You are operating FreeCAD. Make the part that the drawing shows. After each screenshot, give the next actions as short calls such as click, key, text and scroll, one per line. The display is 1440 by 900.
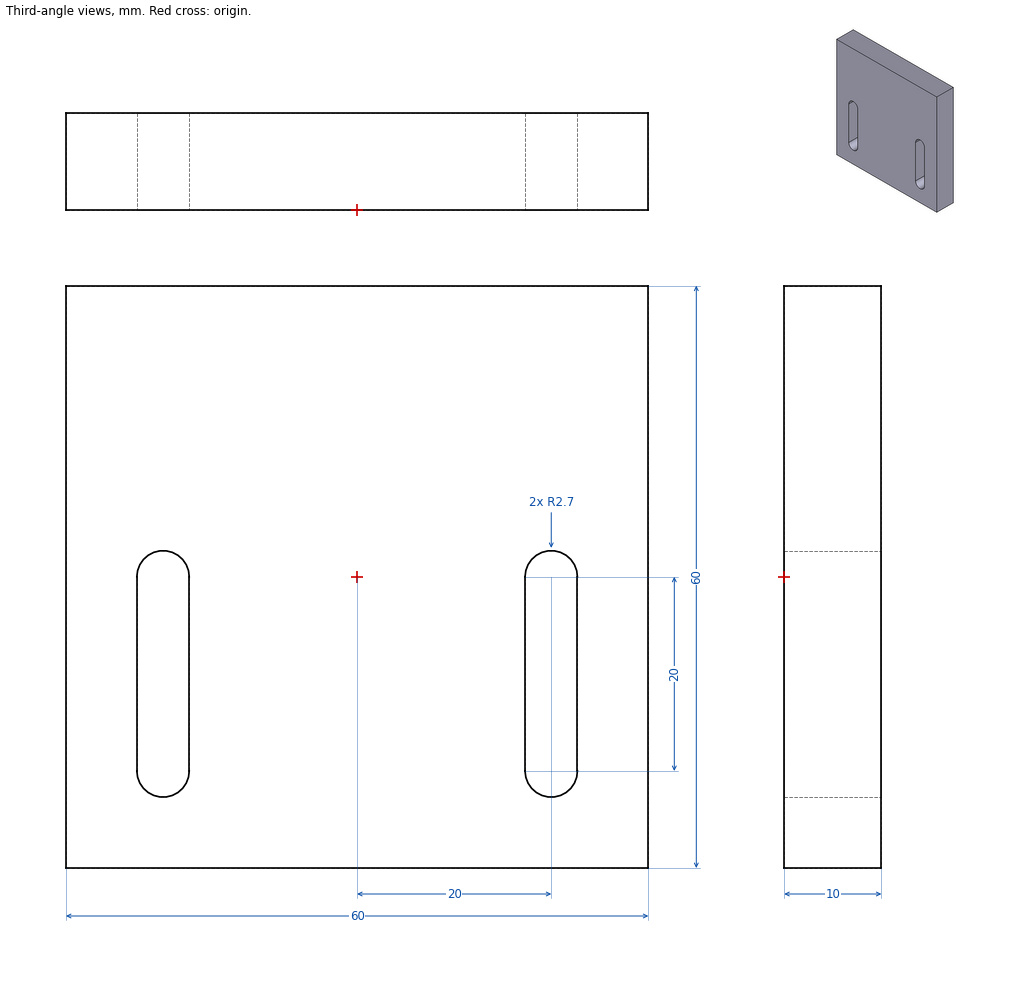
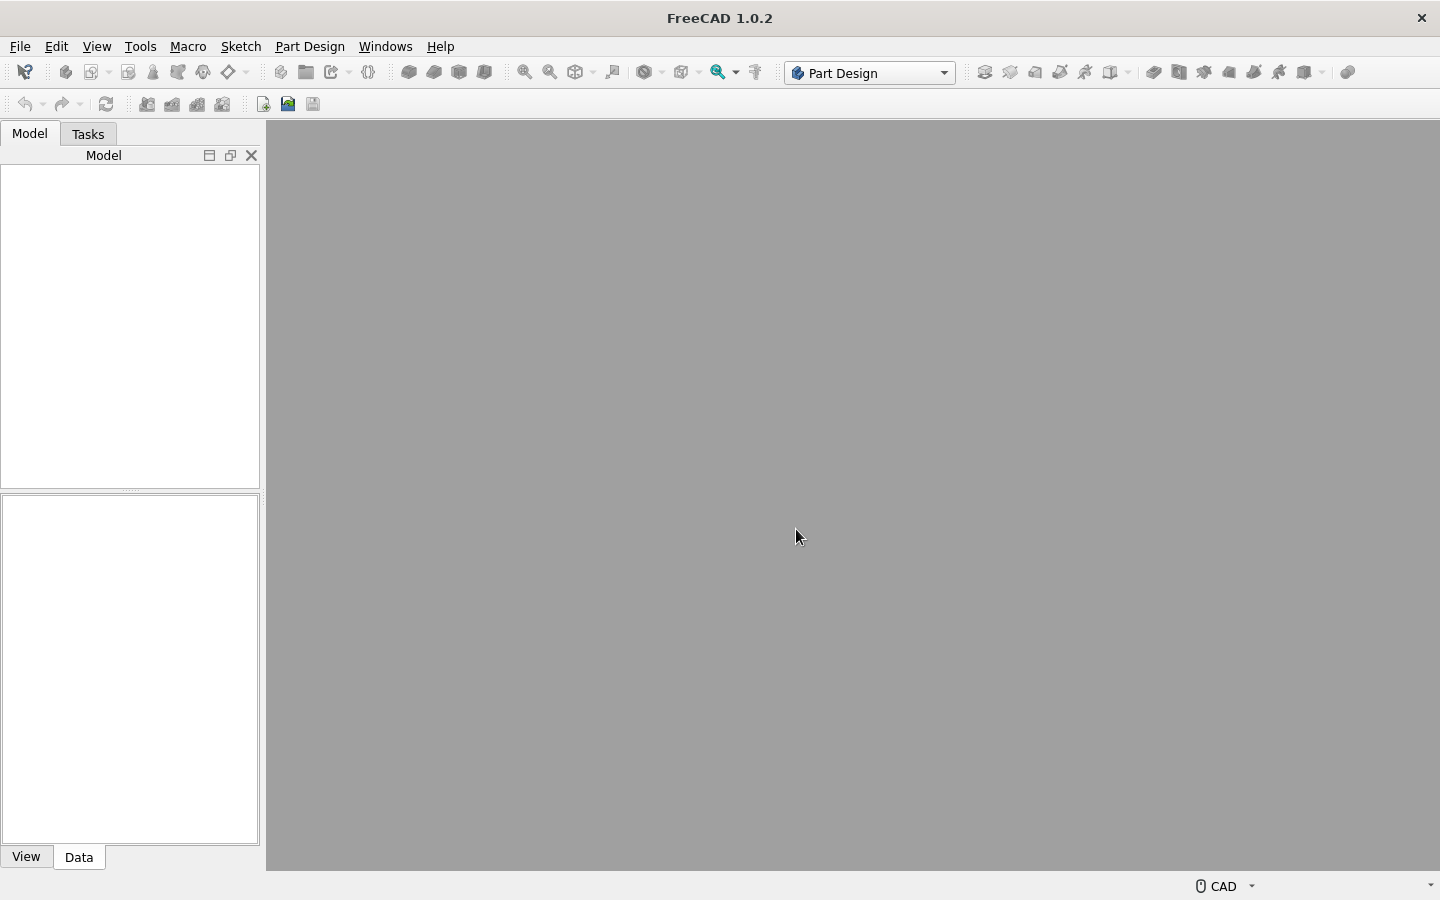
key(ctrl+n)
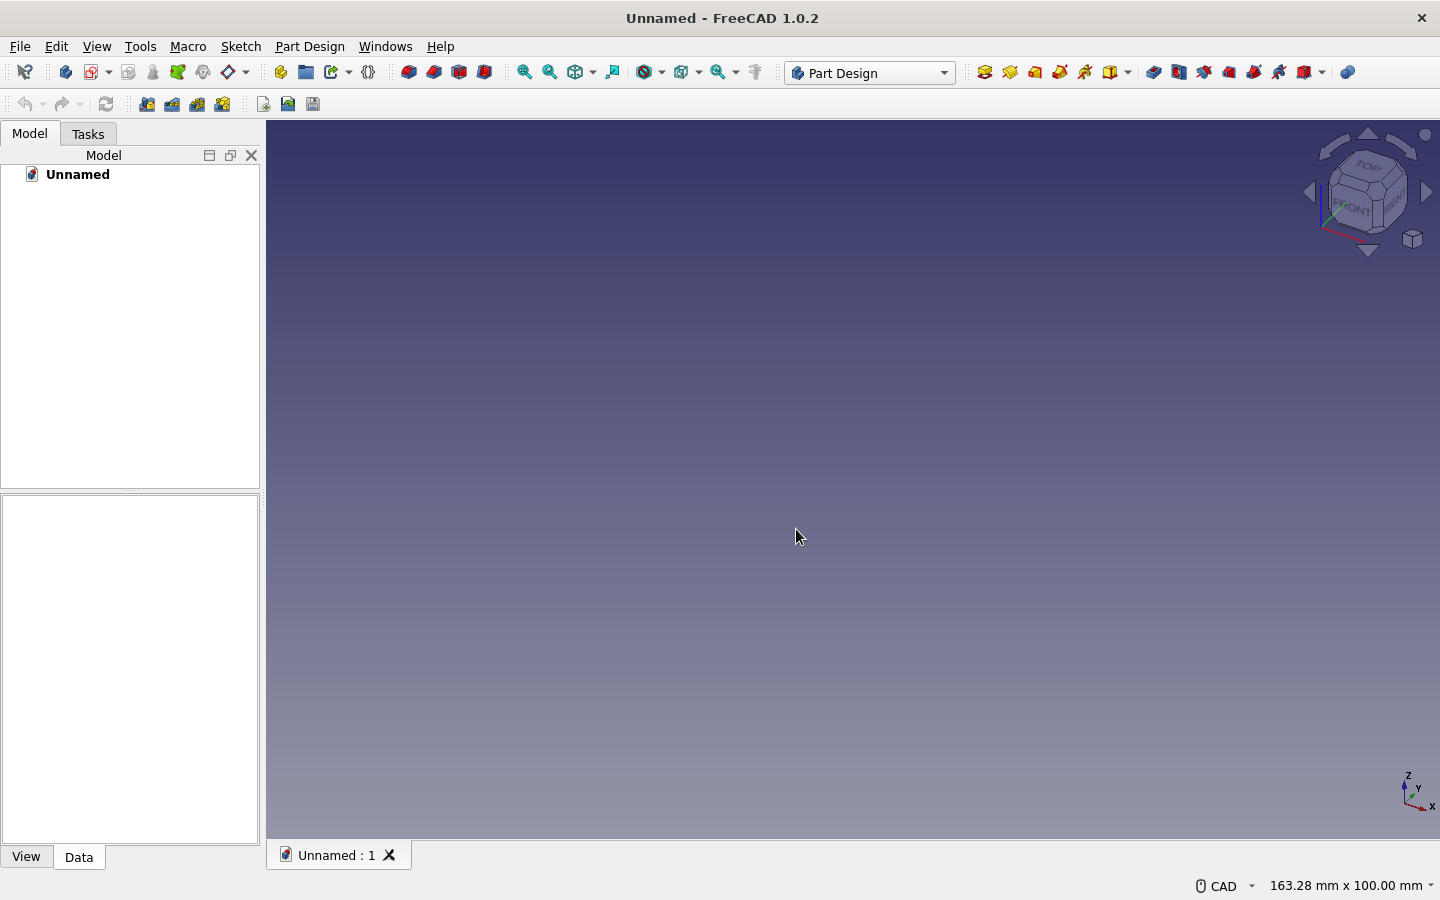
click(90, 72)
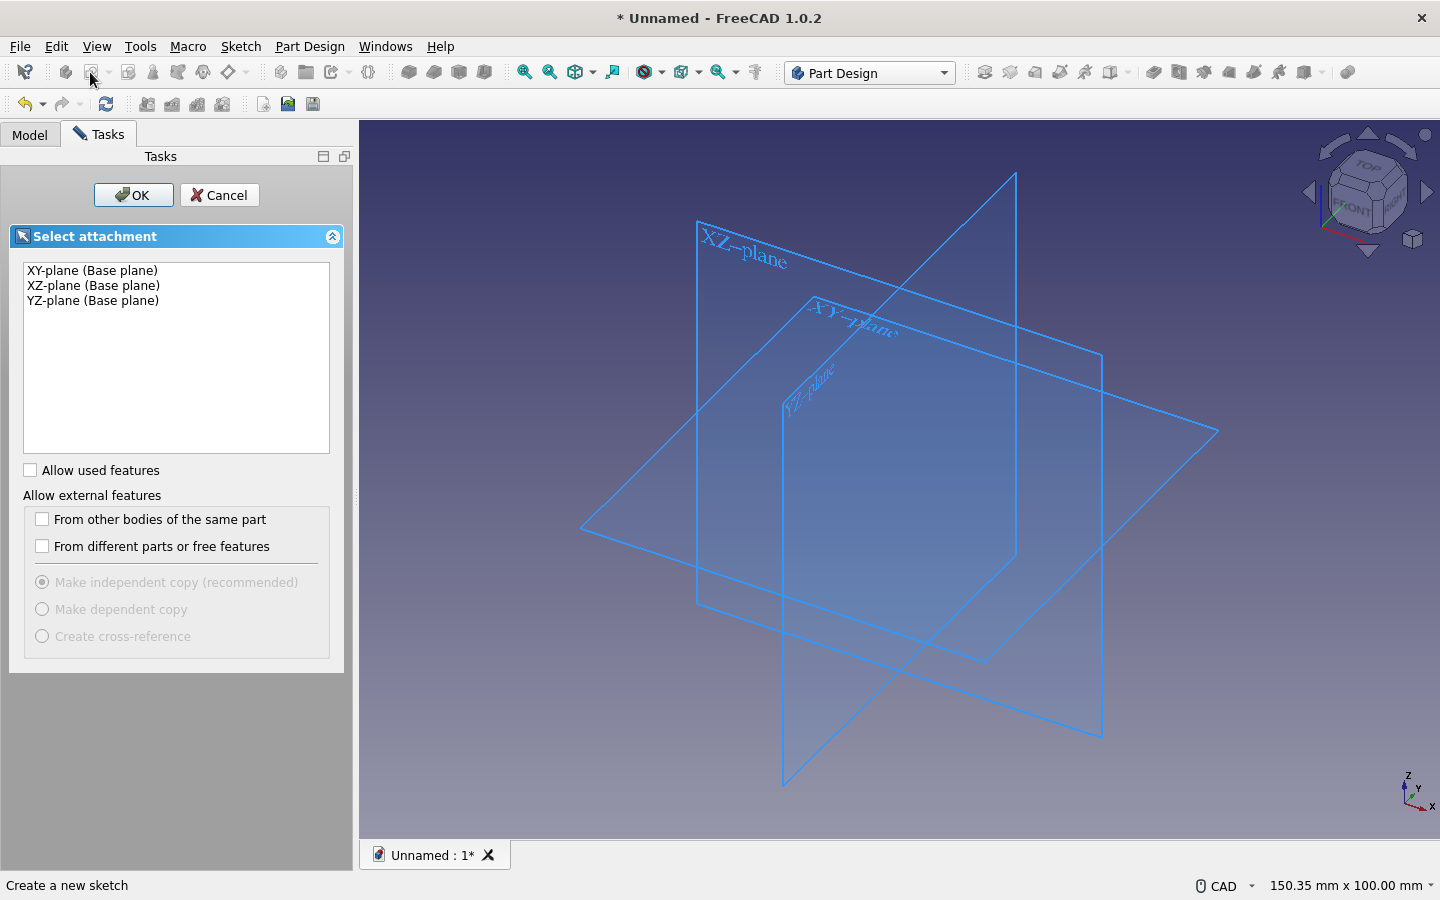
click(84, 286)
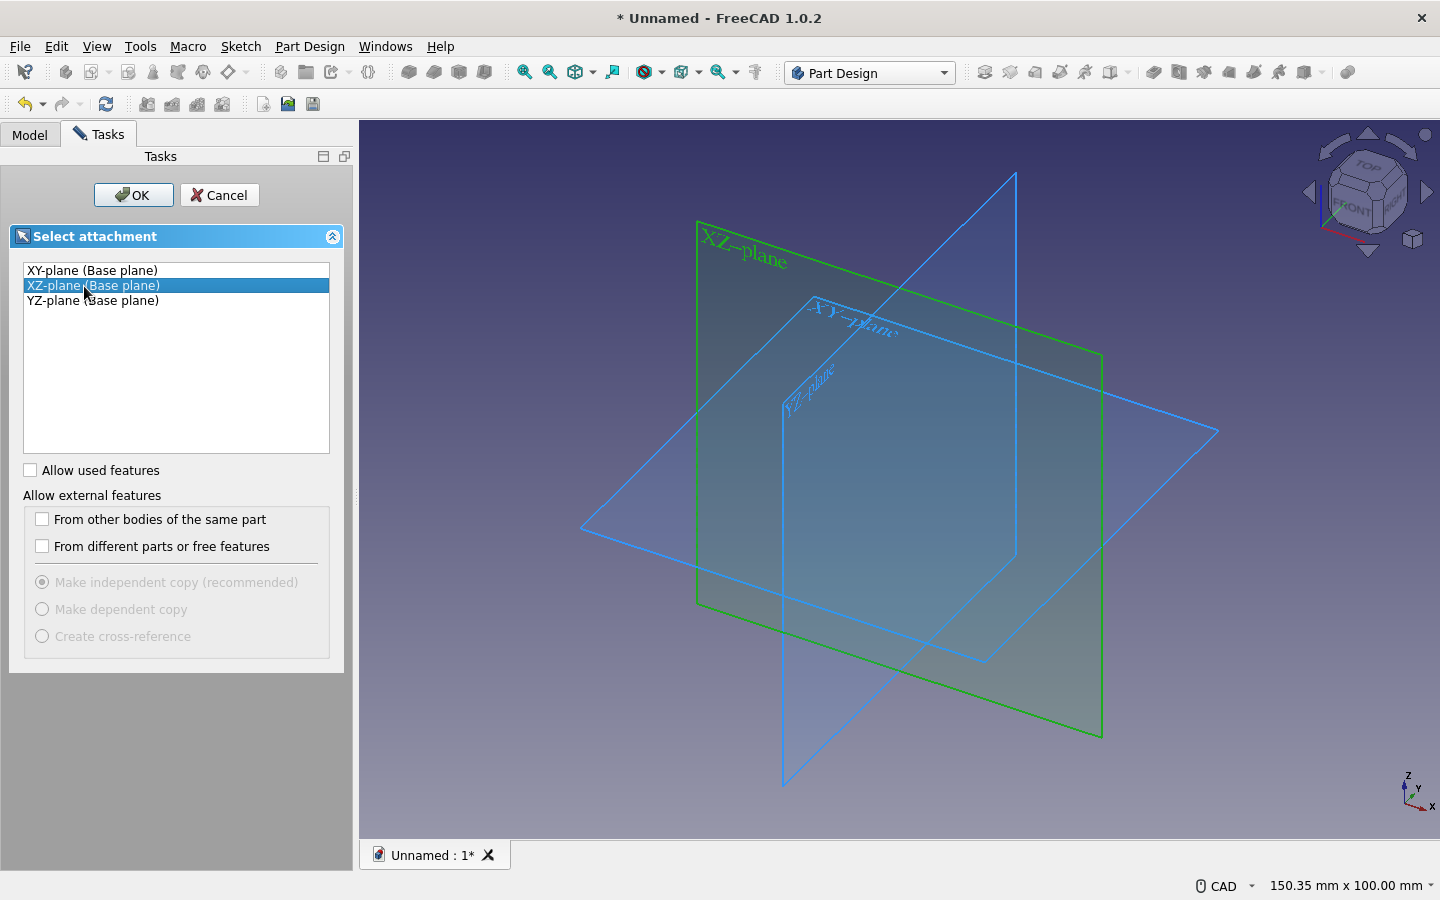
click(134, 195)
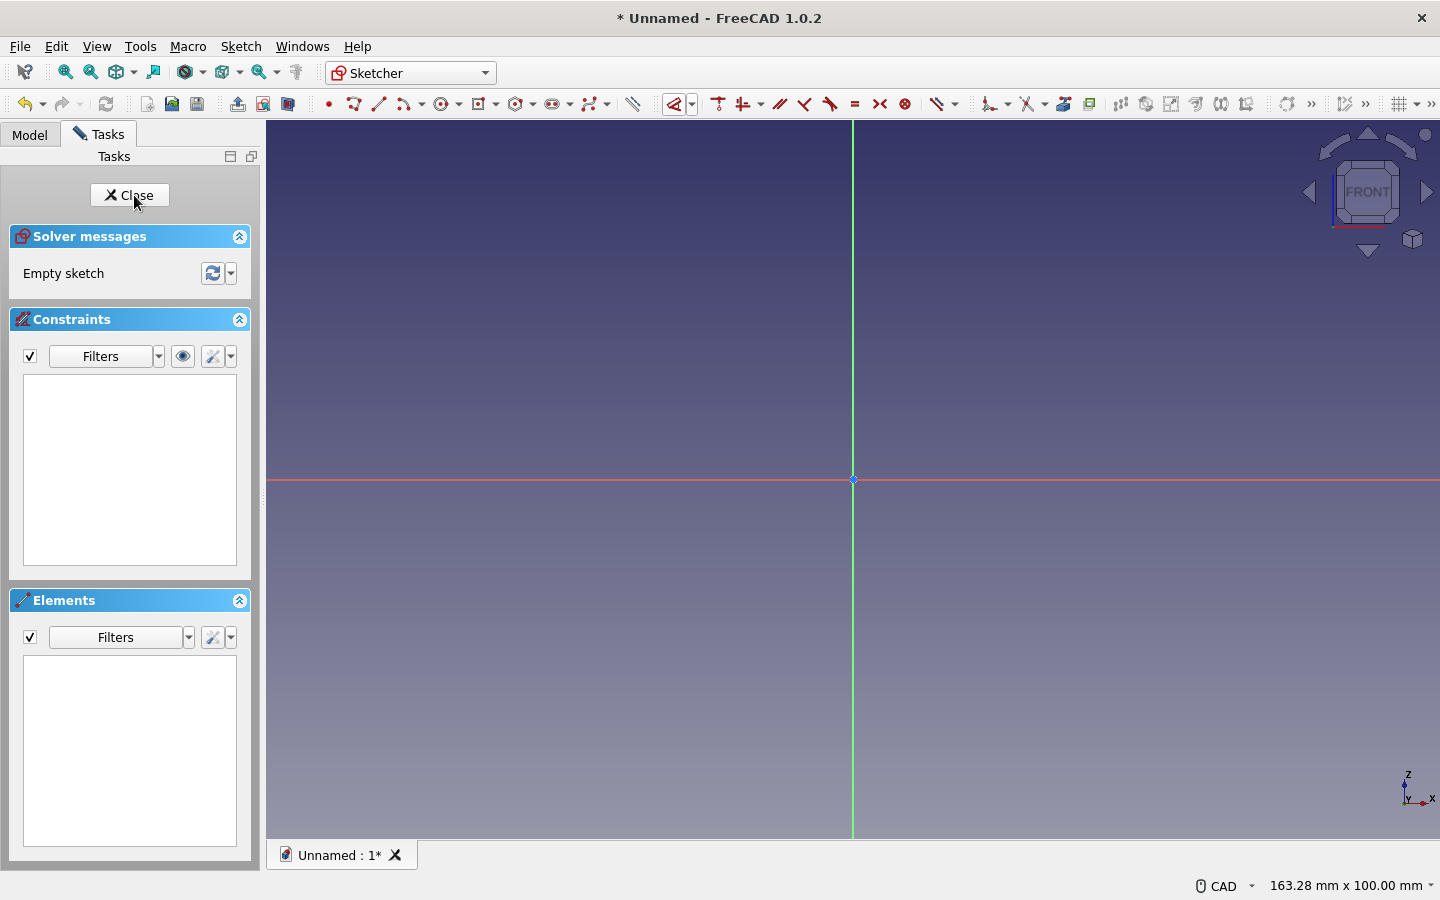
click(478, 104)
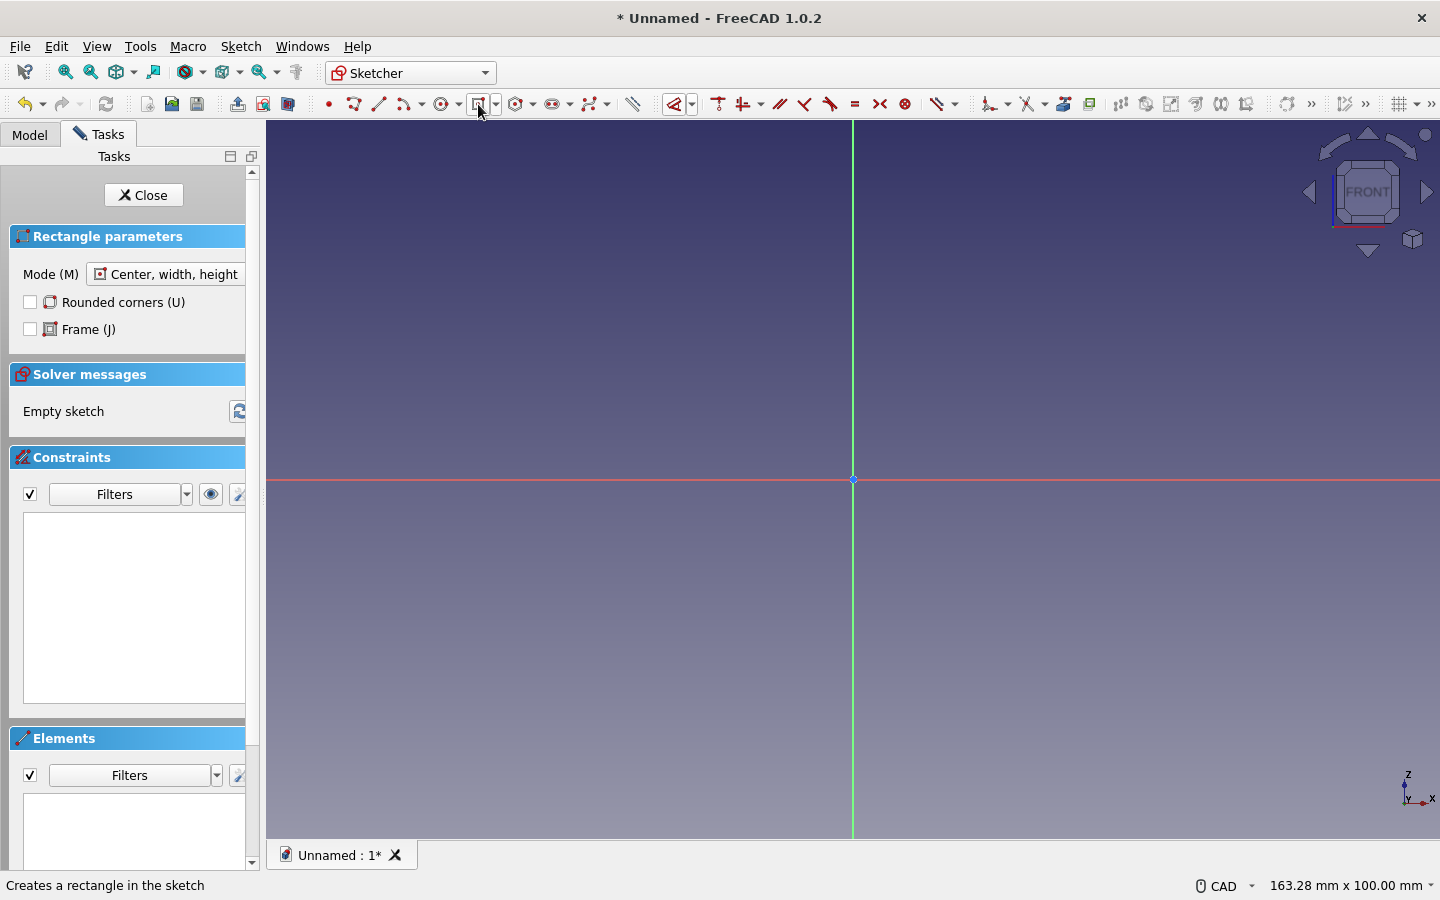
click(853, 480)
click(1069, 264)
key(Escape)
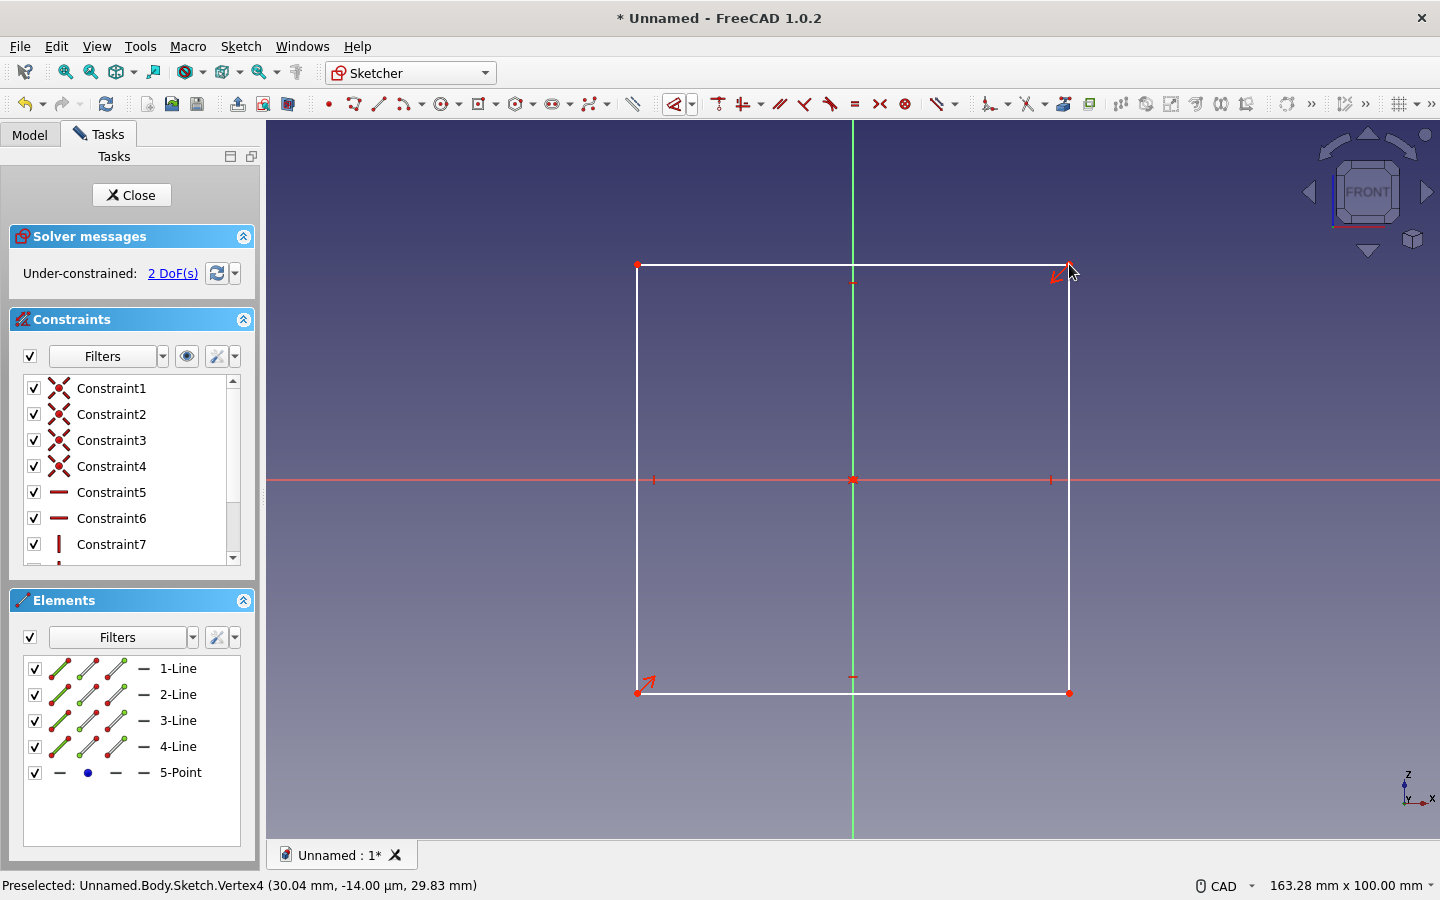
click(767, 694)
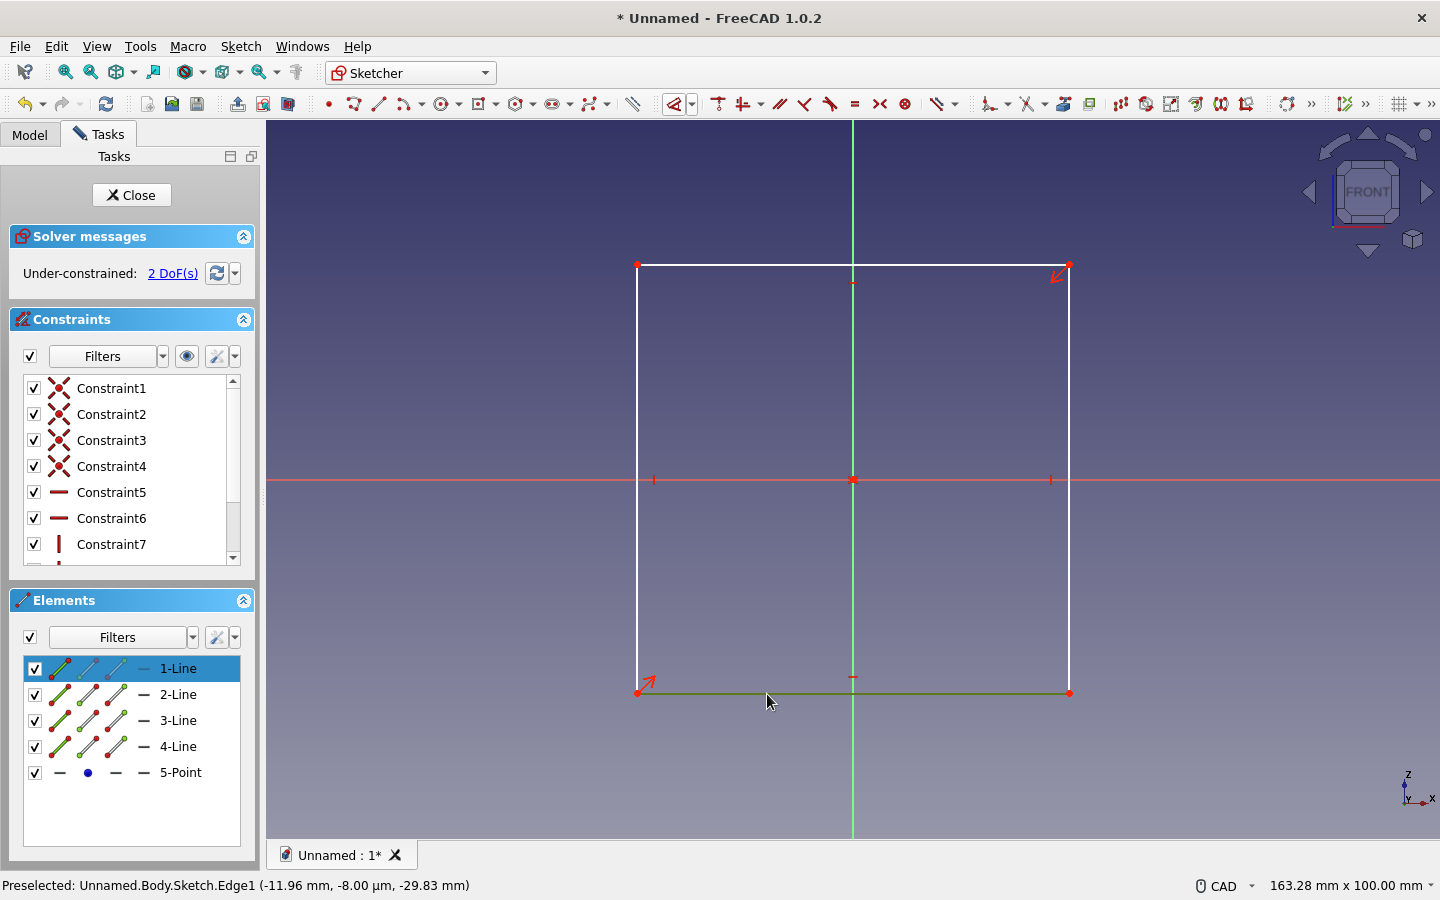
key(l)